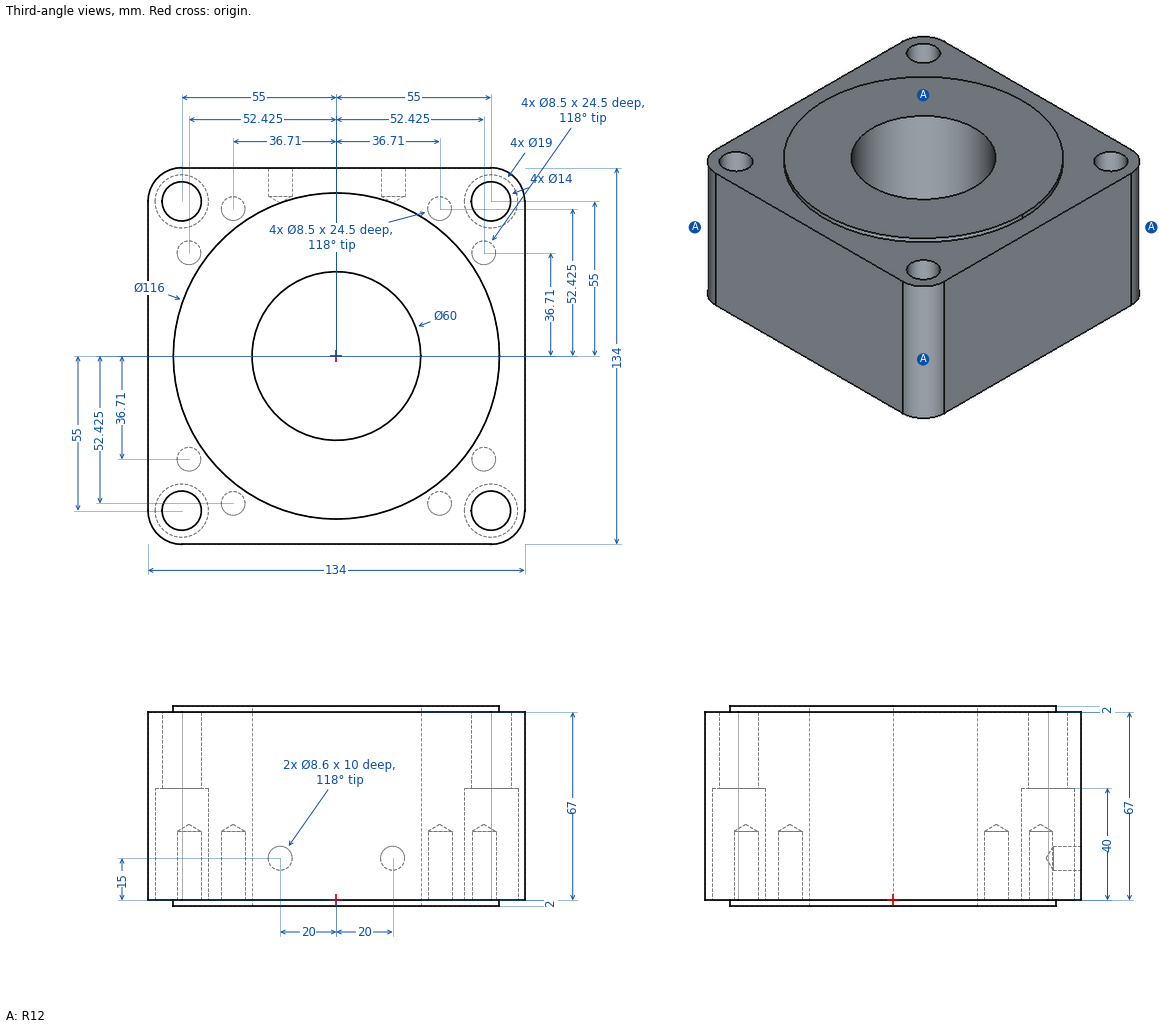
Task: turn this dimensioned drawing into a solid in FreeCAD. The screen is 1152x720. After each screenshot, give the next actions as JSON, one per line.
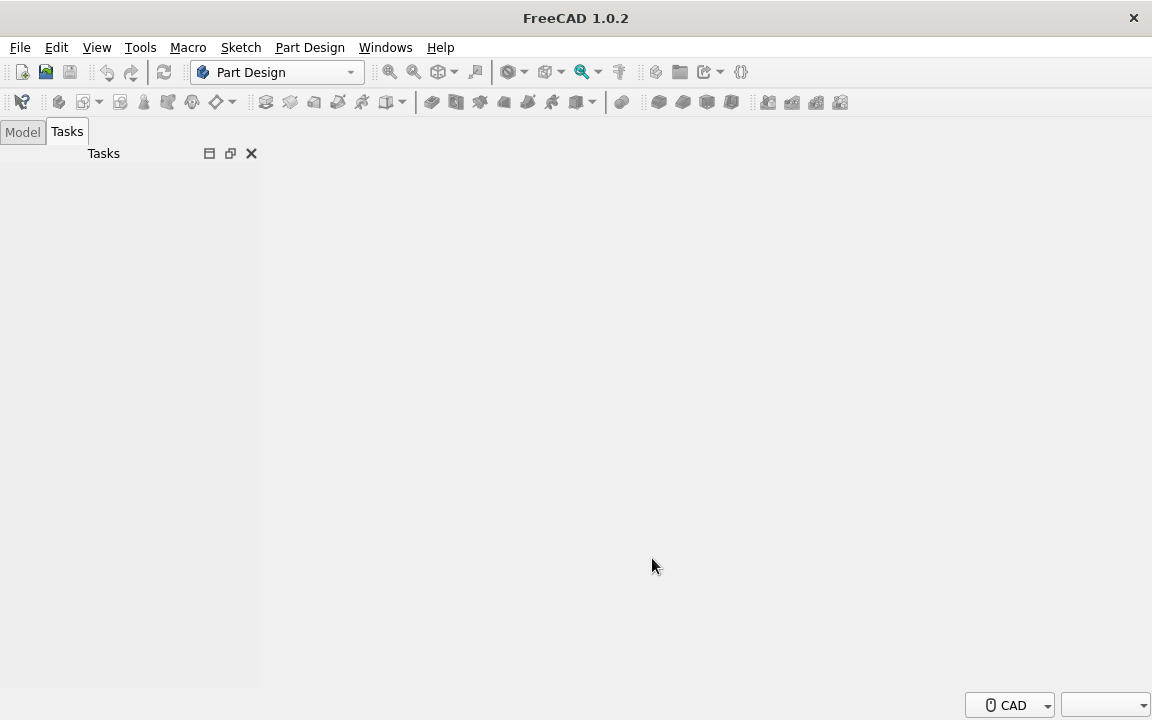
{"action": "left_click", "coordinate": [22, 72]}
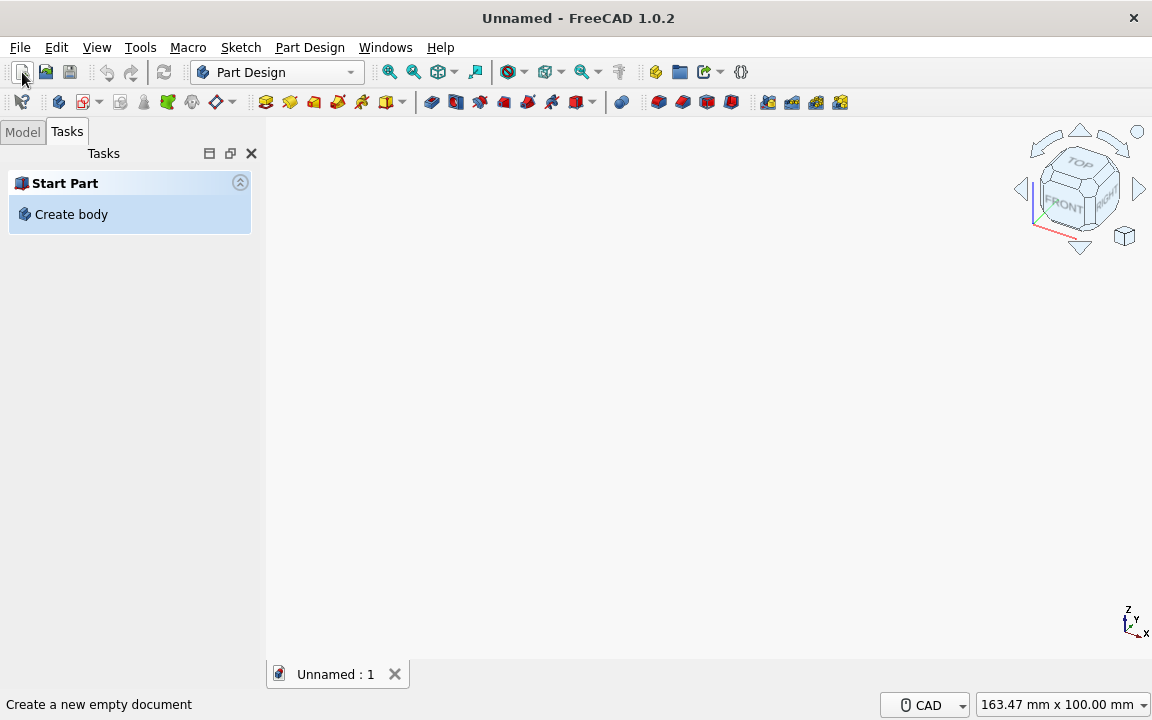
{"action": "left_click", "coordinate": [84, 102]}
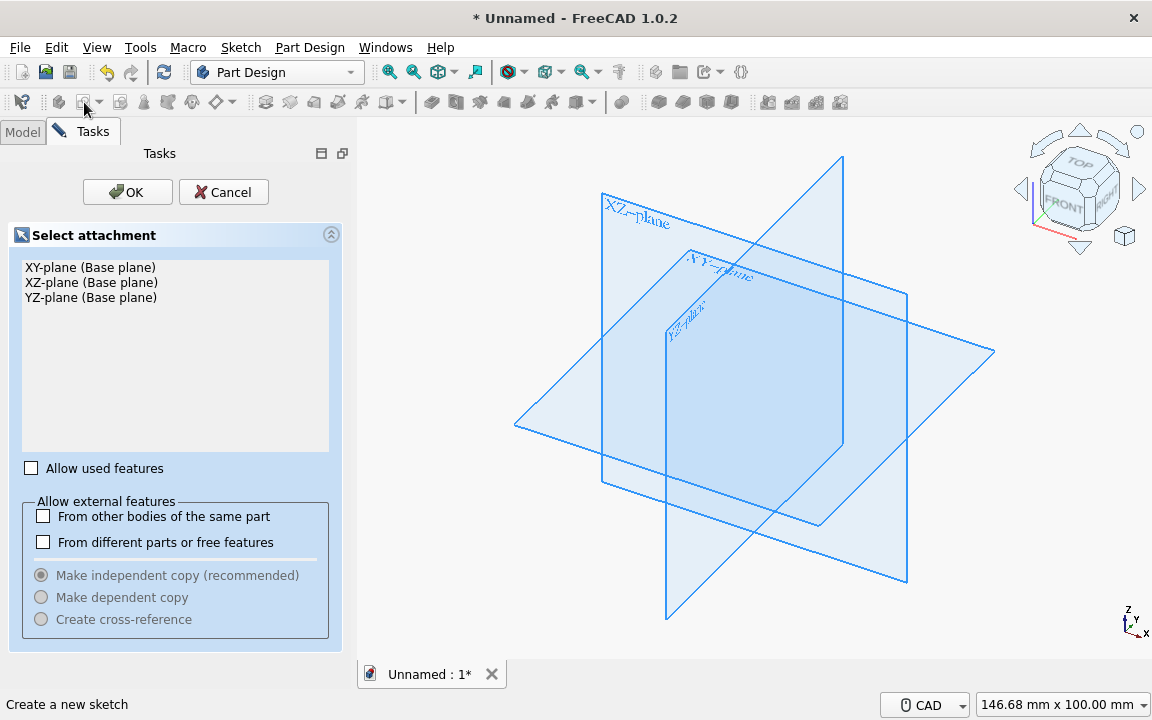
{"action": "left_click", "coordinate": [82, 268]}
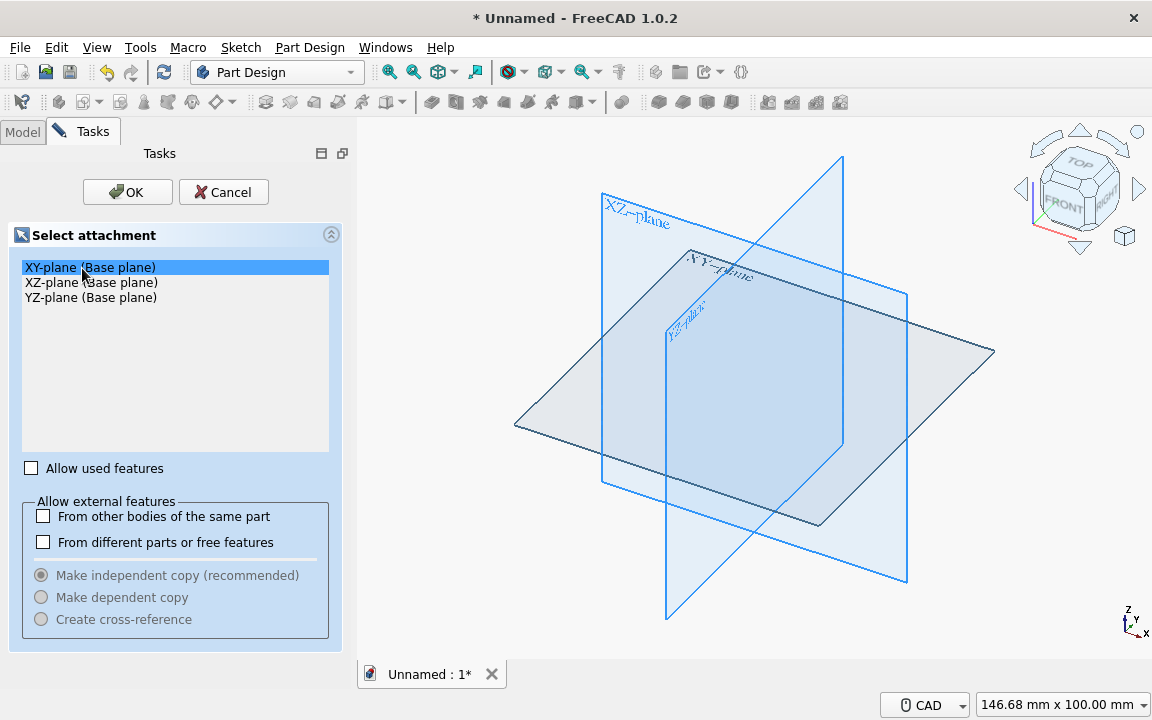
{"action": "left_click", "coordinate": [128, 192]}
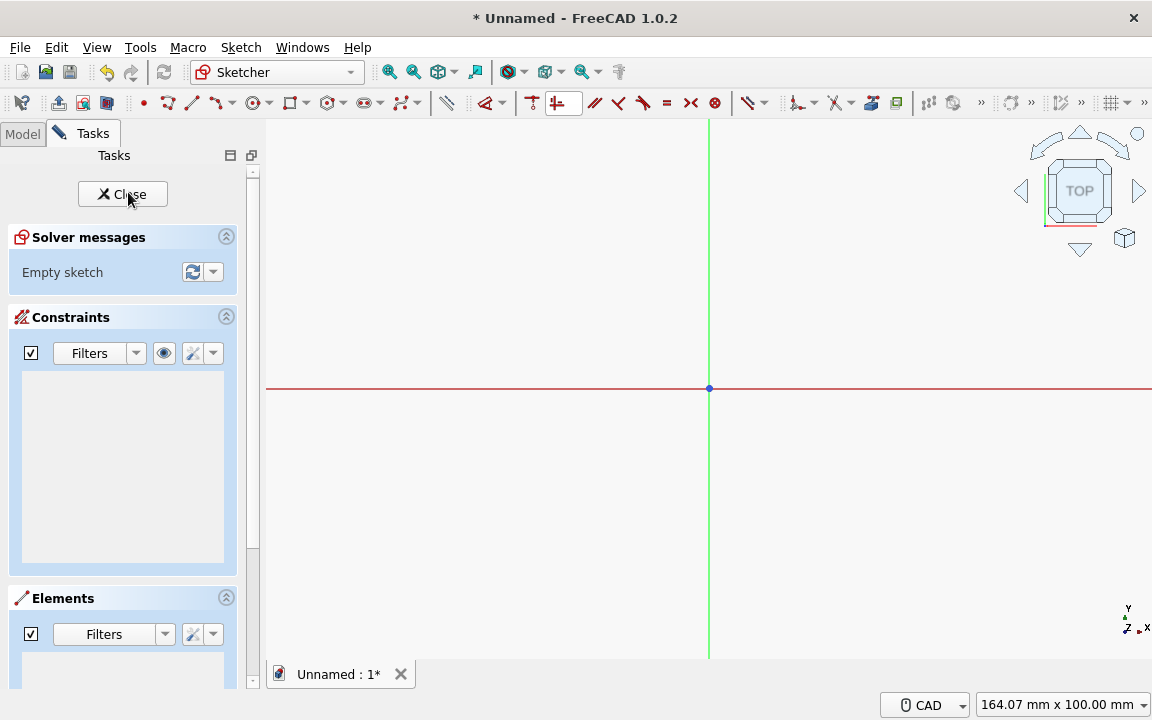
{"action": "scroll", "coordinate": [585, 389], "scroll_direction": "down", "scroll_amount": 4}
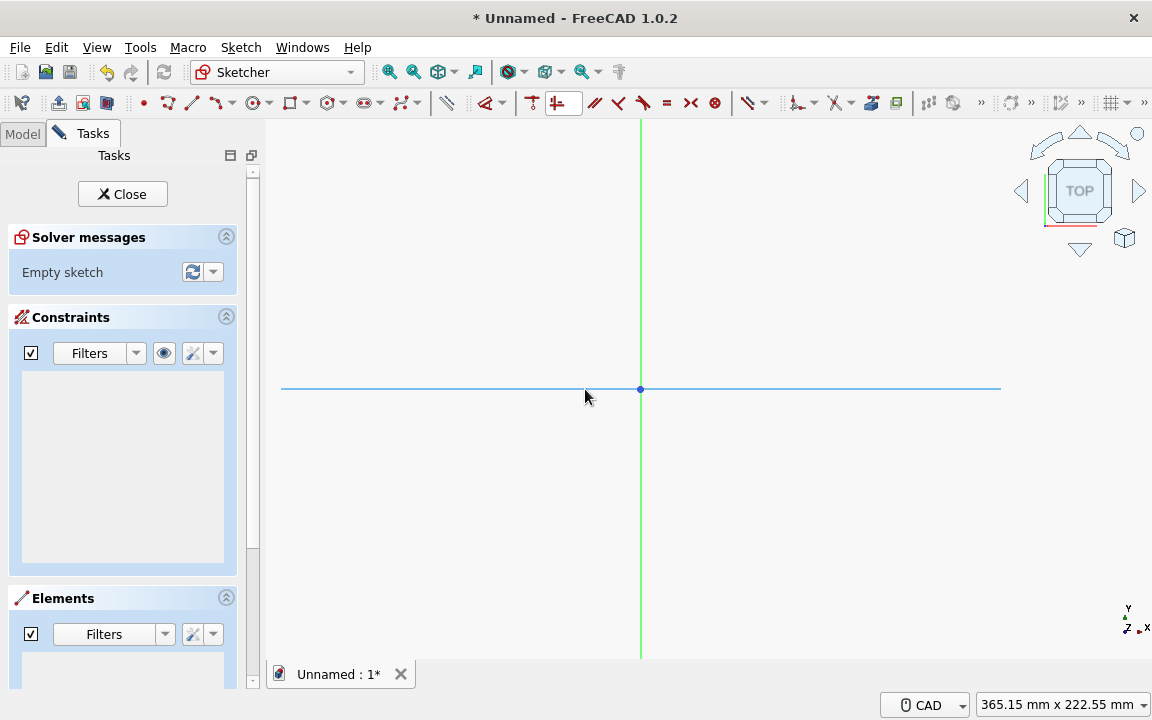
{"action": "left_click", "coordinate": [308, 104]}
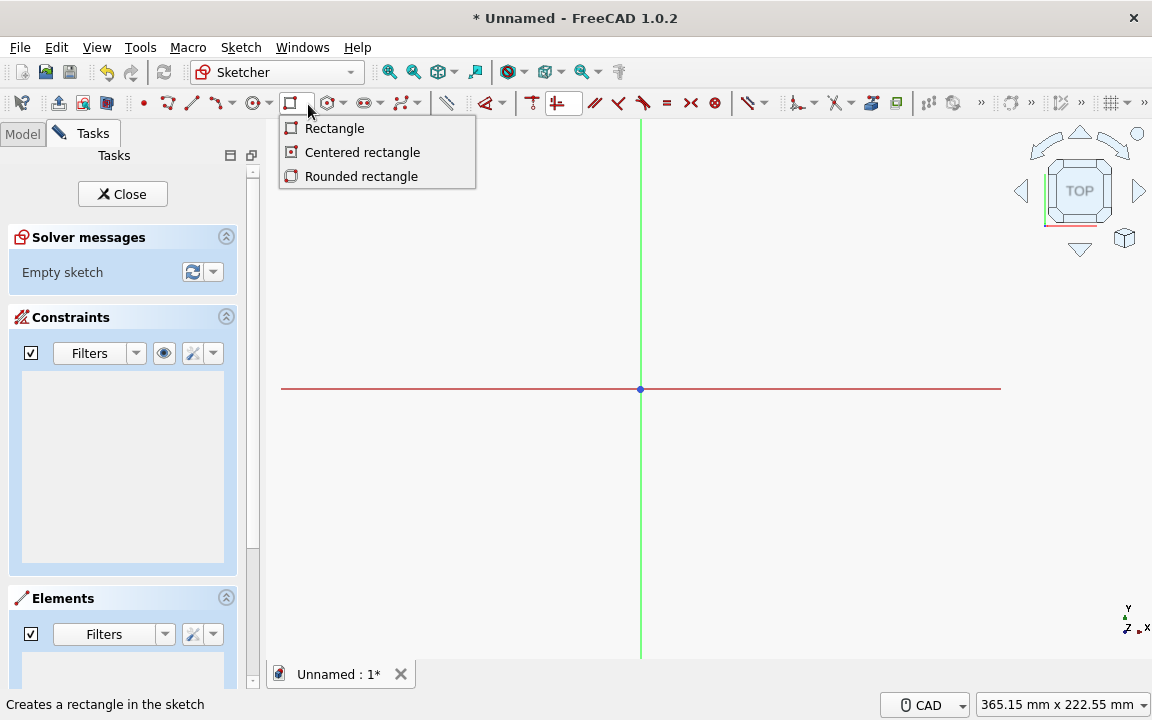
{"action": "left_click", "coordinate": [378, 152]}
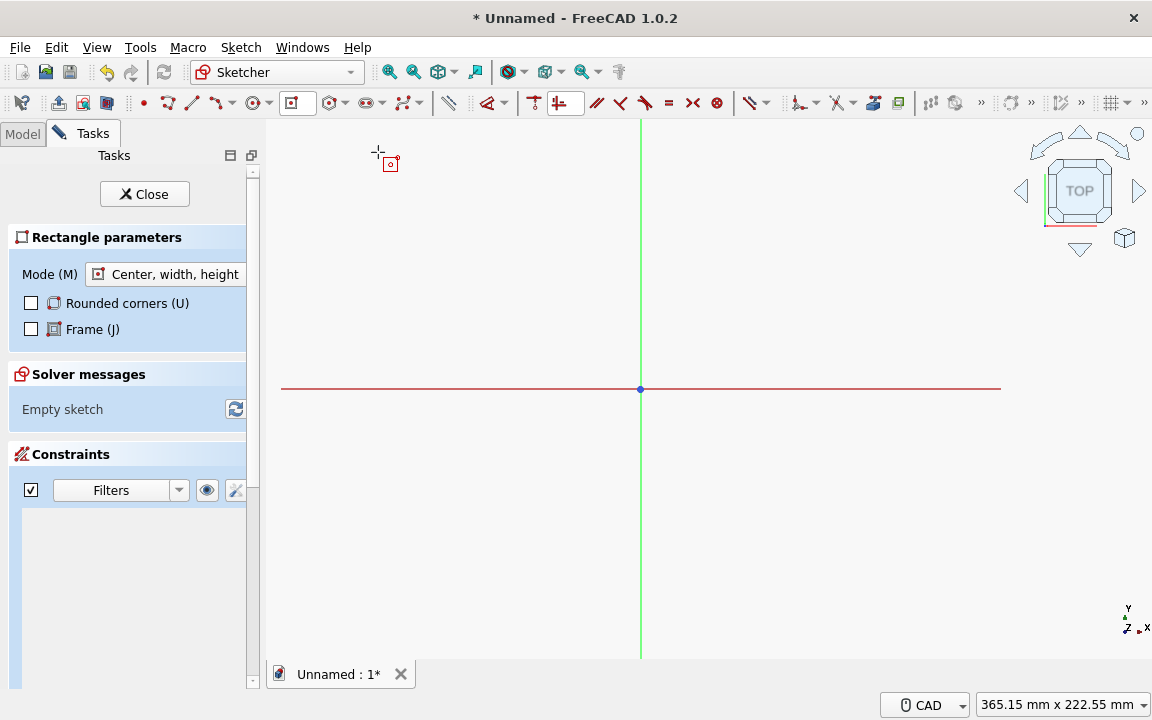
{"action": "left_click", "coordinate": [641, 389]}
{"action": "left_click", "coordinate": [803, 227]}
{"action": "key", "text": "Escape"}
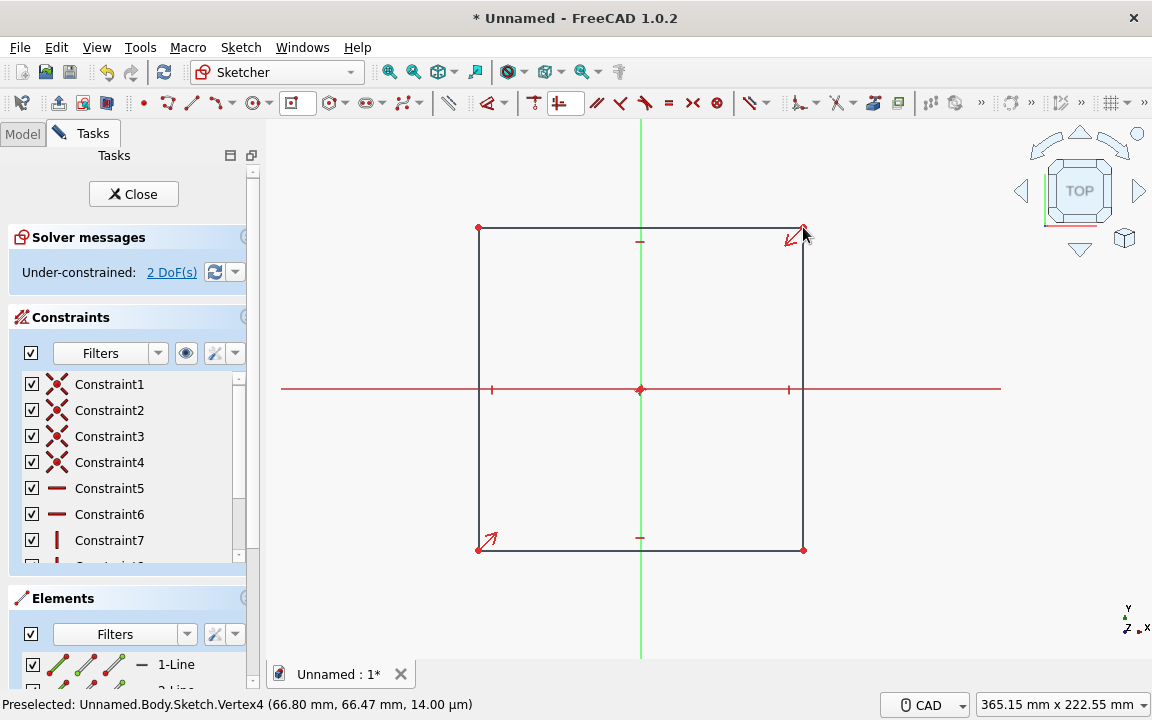
{"action": "left_click", "coordinate": [576, 551]}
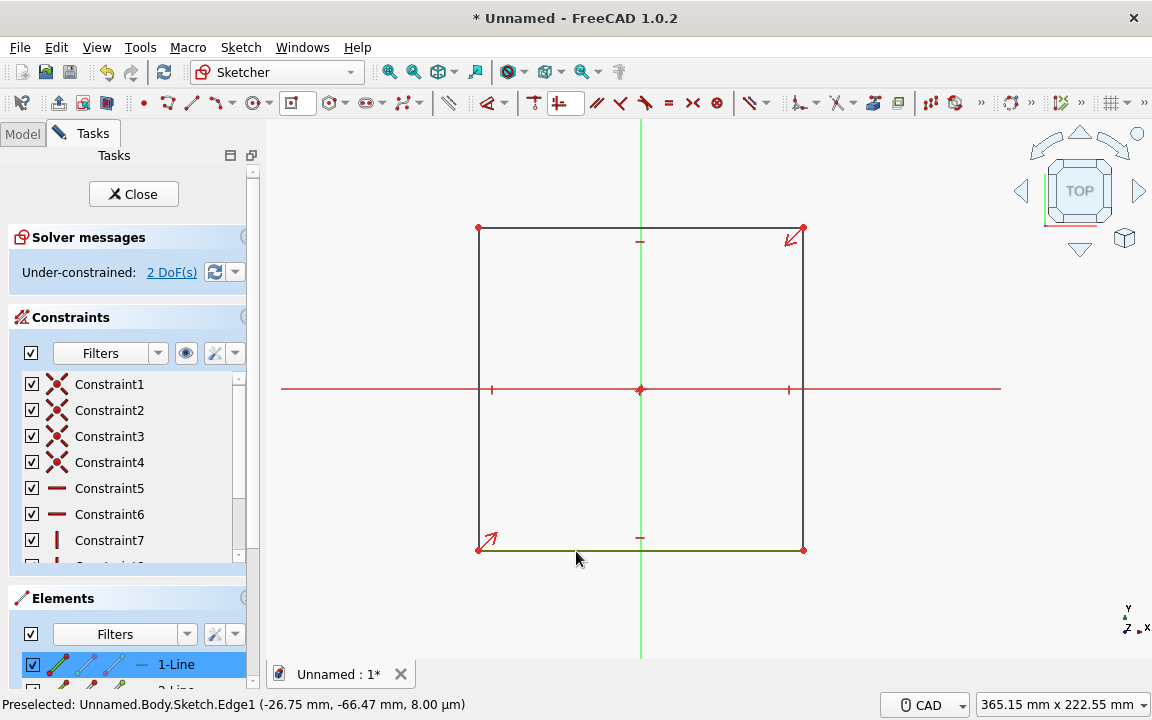
{"action": "left_click", "coordinate": [506, 104]}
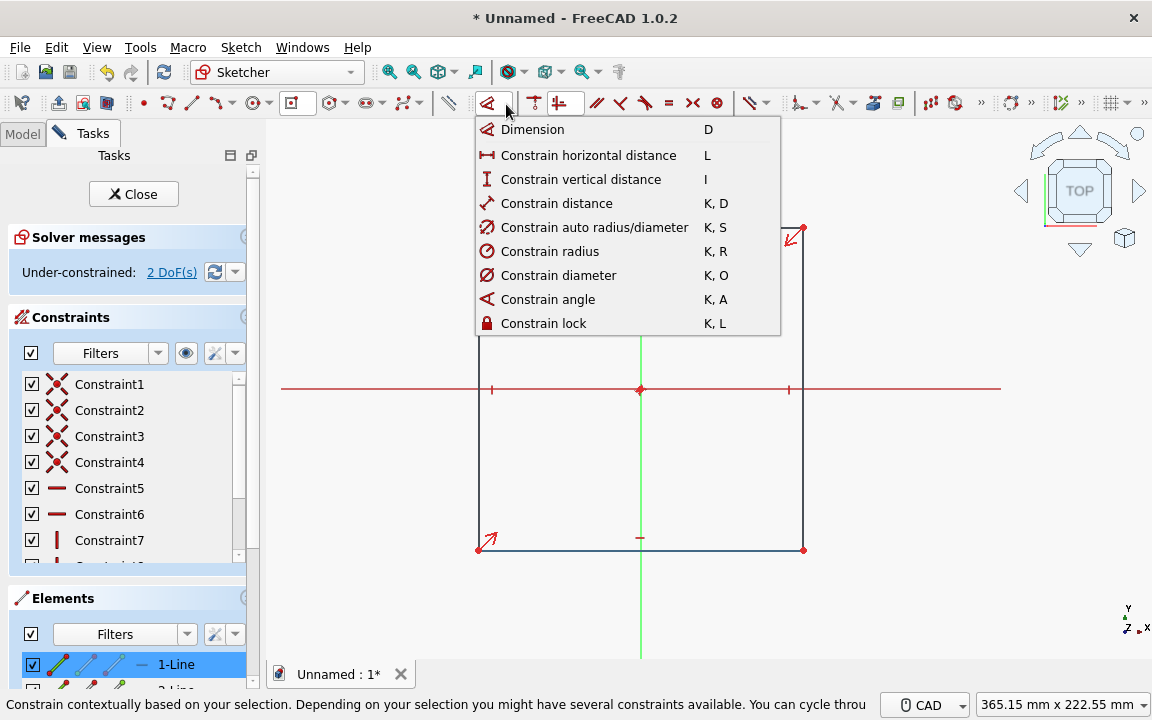
{"action": "left_click", "coordinate": [628, 155]}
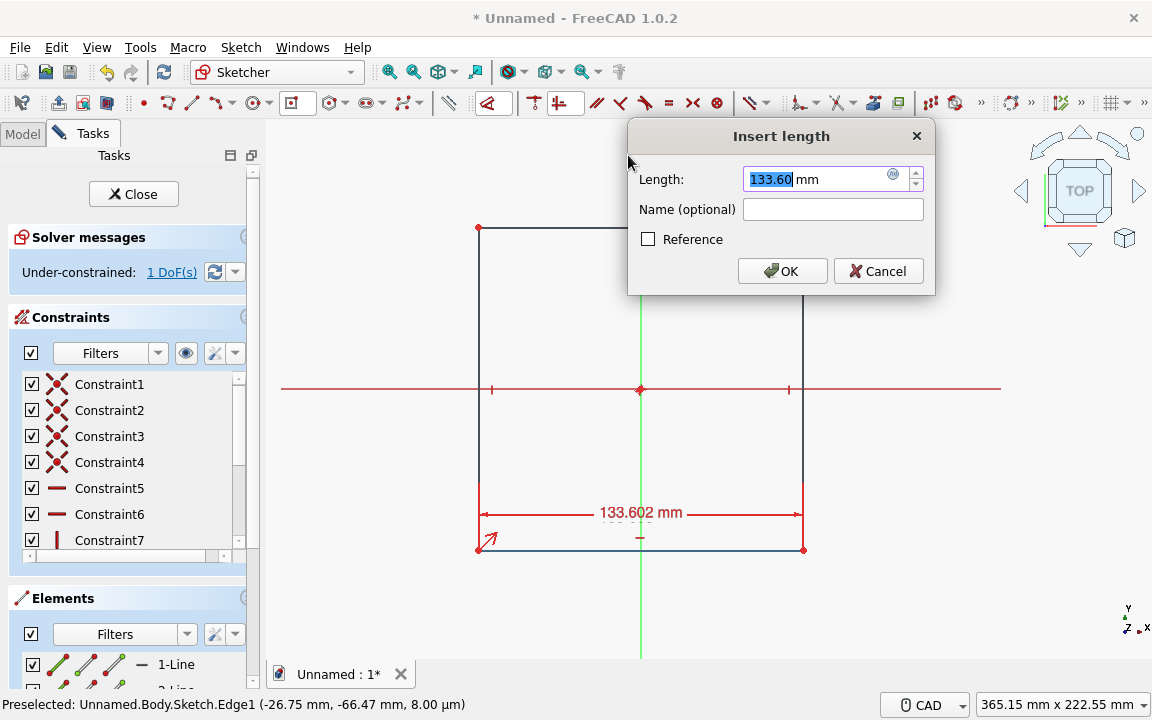
{"action": "type", "text": "134"}
{"action": "key", "text": "Return"}